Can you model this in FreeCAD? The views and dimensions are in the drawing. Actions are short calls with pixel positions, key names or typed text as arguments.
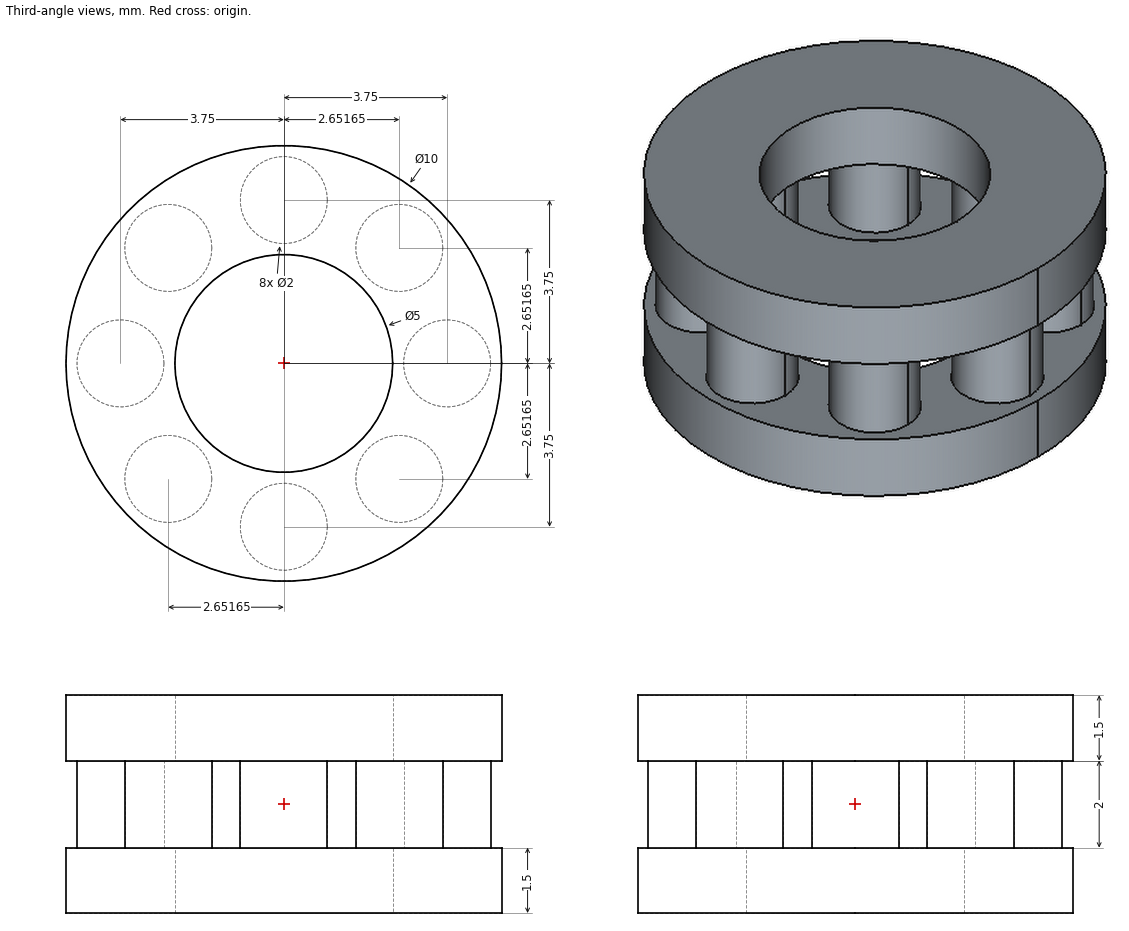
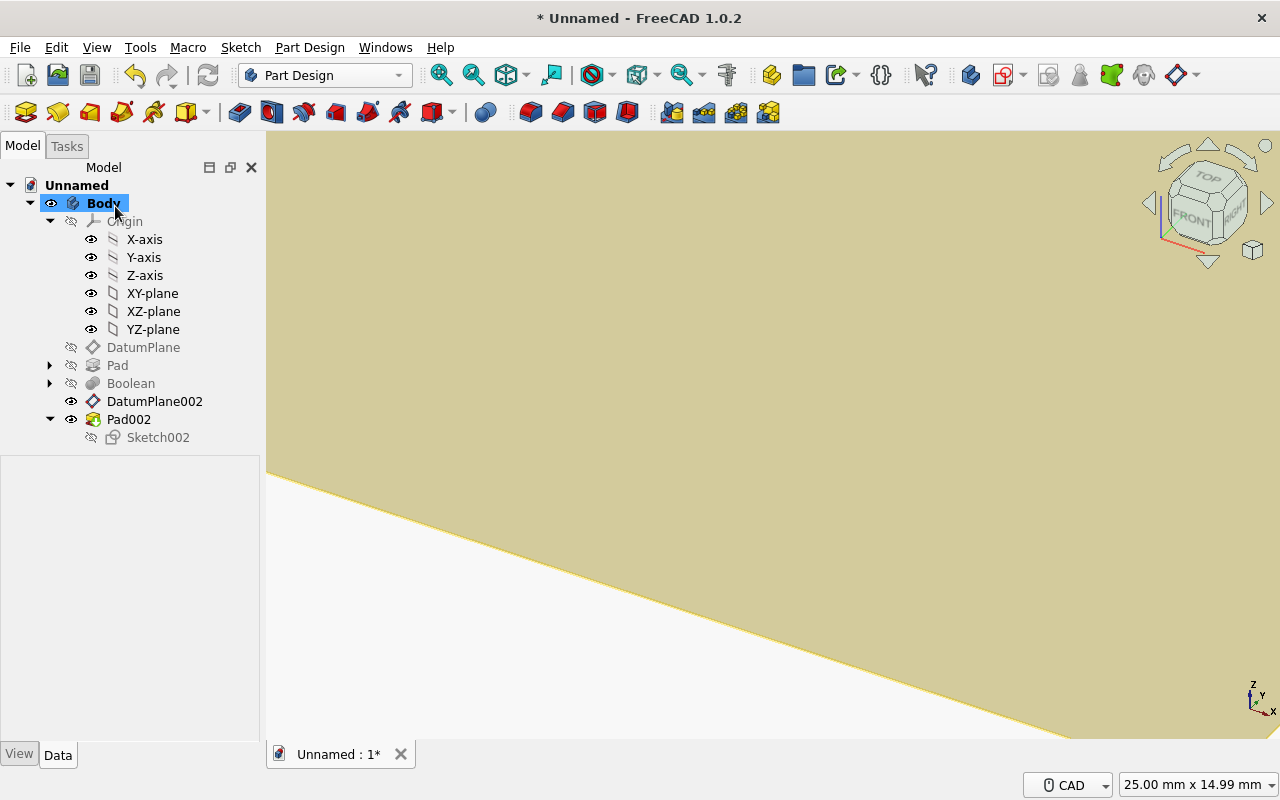
click(116, 401)
key(space)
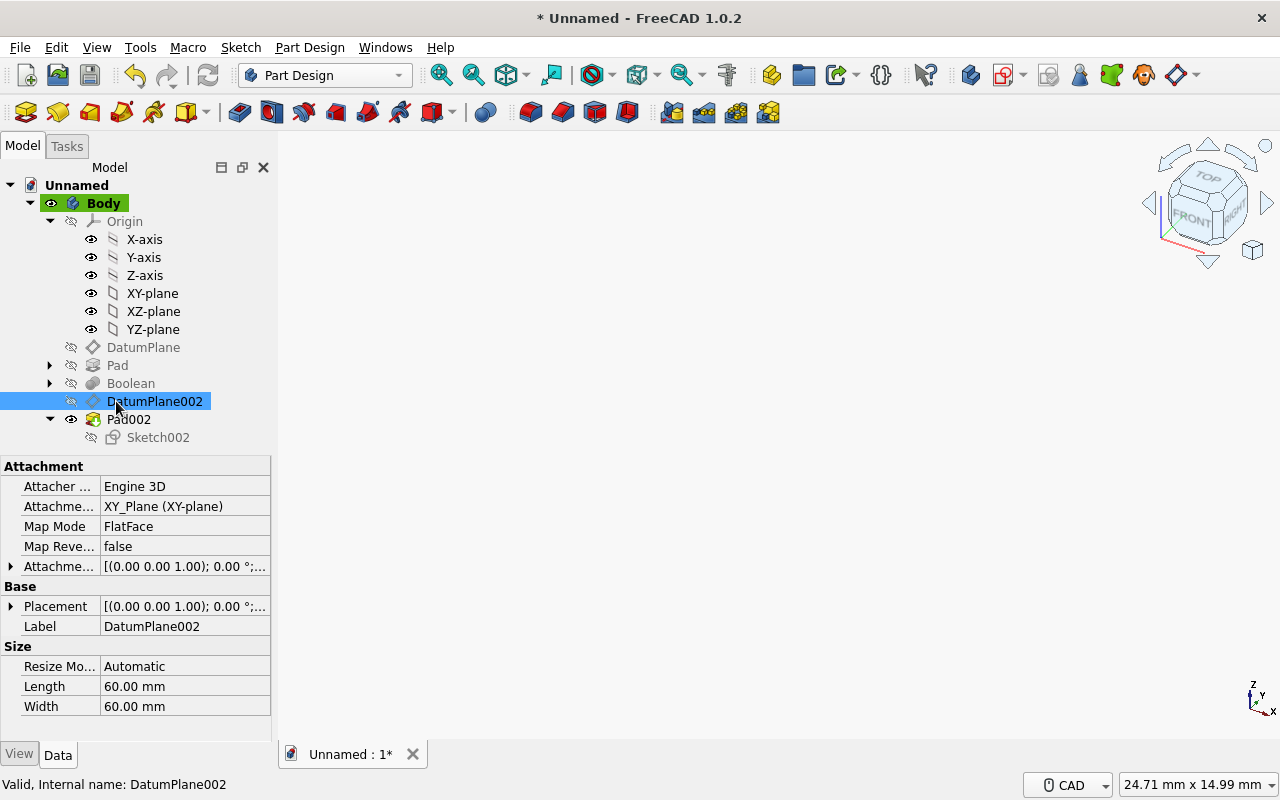
key(0)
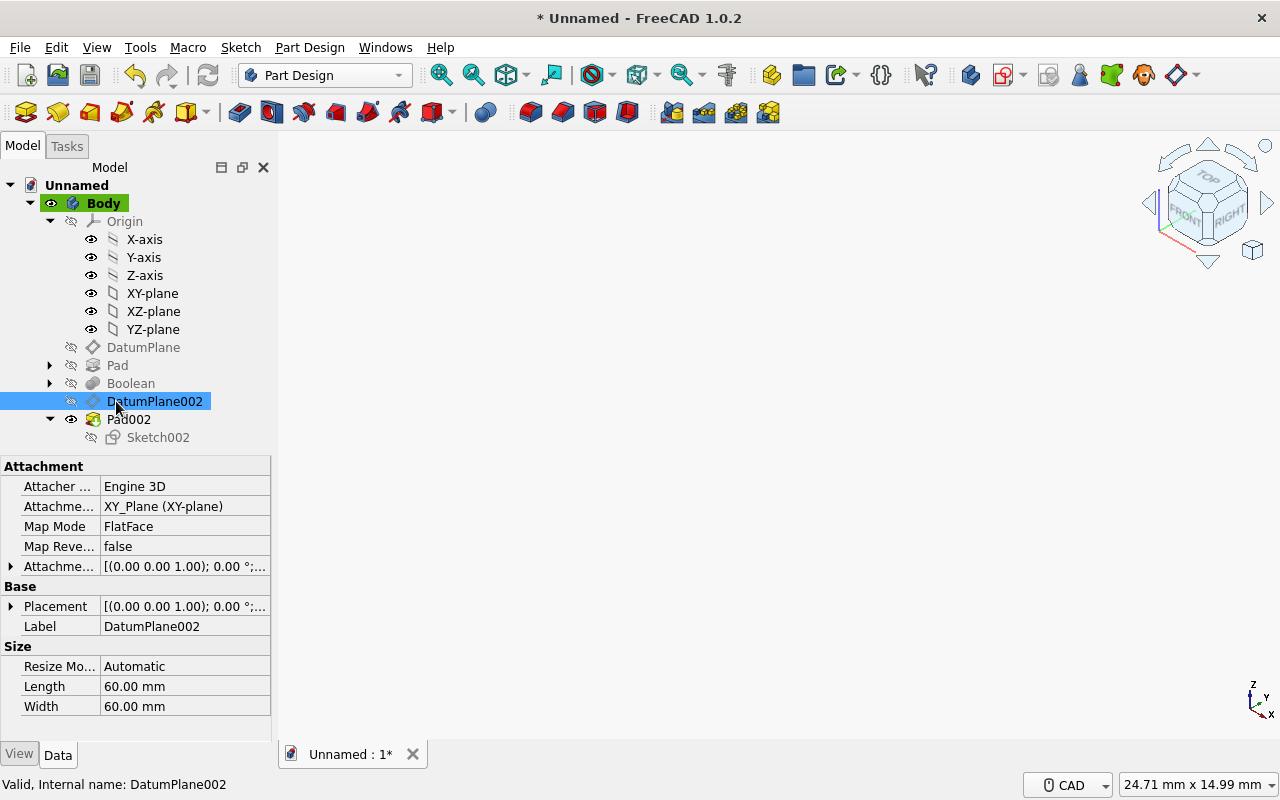
key(v)
key(f)